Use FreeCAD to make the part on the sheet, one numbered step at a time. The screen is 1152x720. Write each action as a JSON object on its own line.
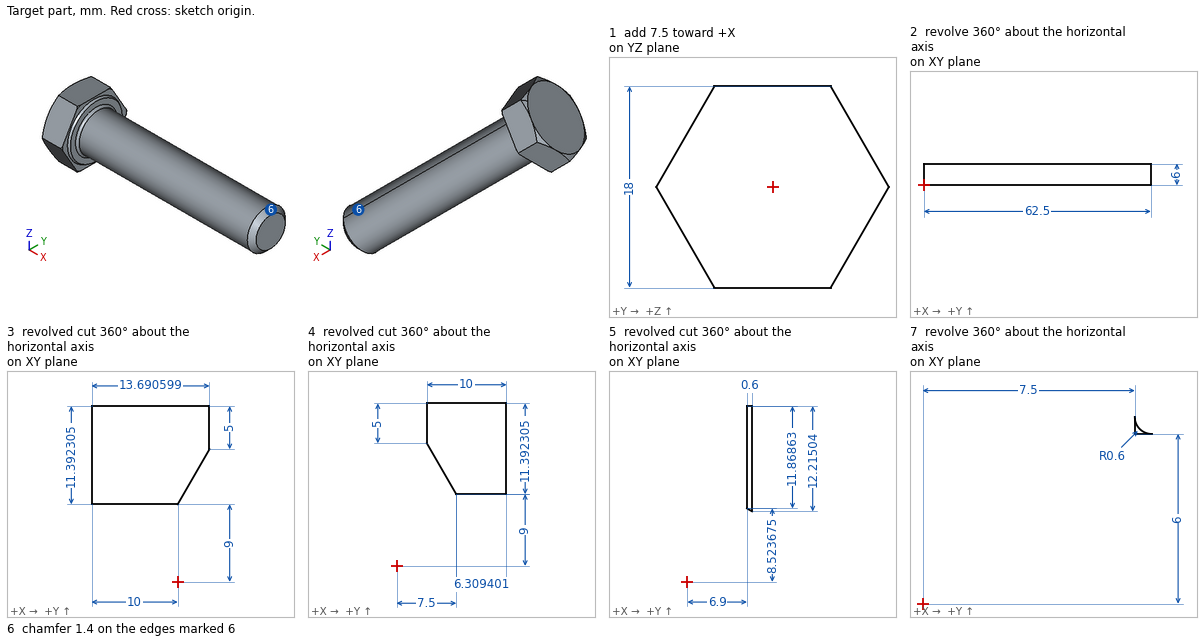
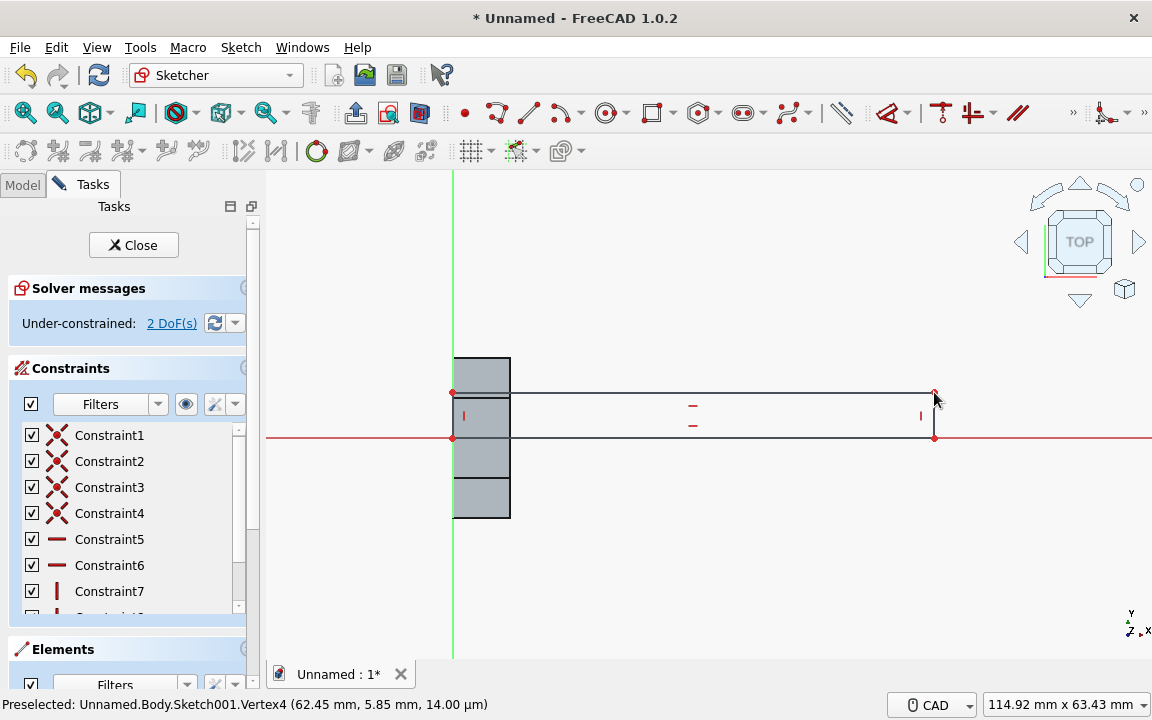
{"action": "key", "text": "d"}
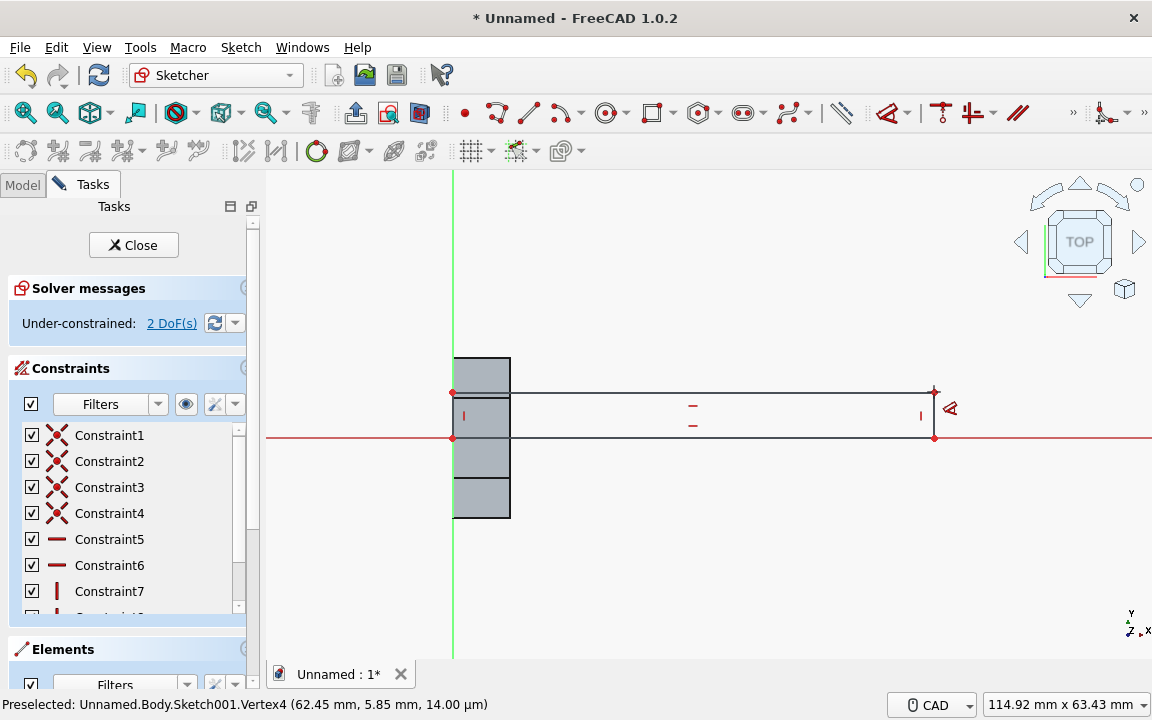
{"action": "left_click", "coordinate": [934, 425]}
{"action": "left_click", "coordinate": [968, 416]}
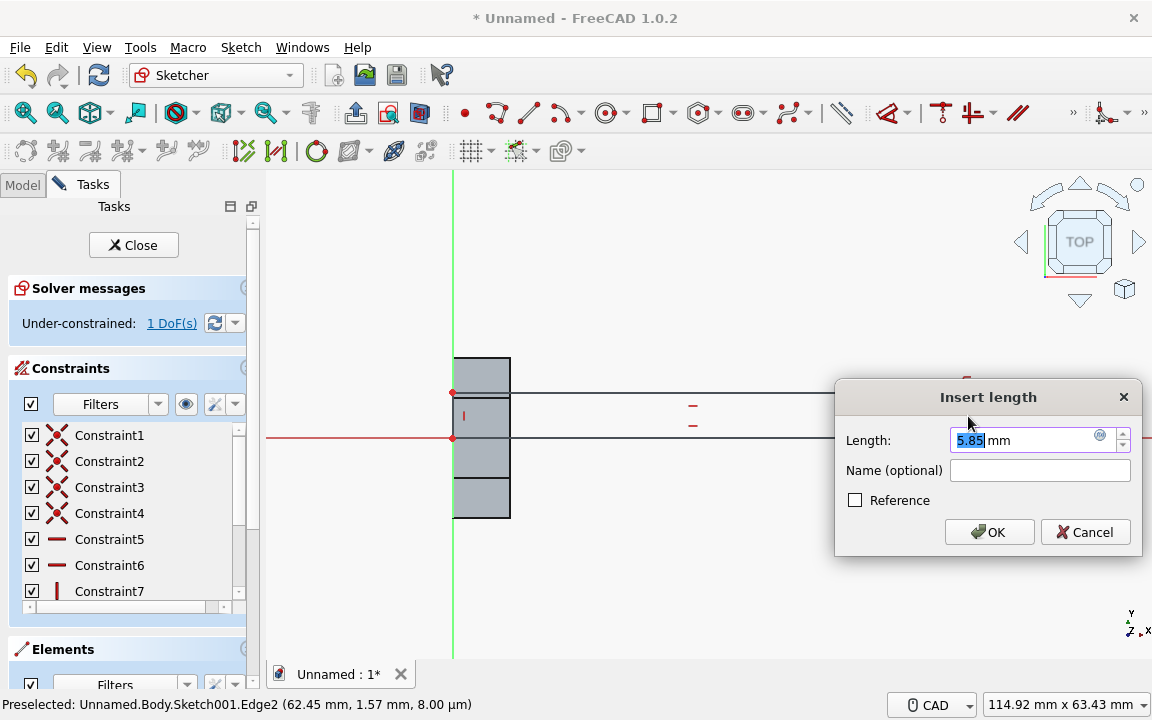
{"action": "type", "text": "6"}
{"action": "key", "text": "Return"}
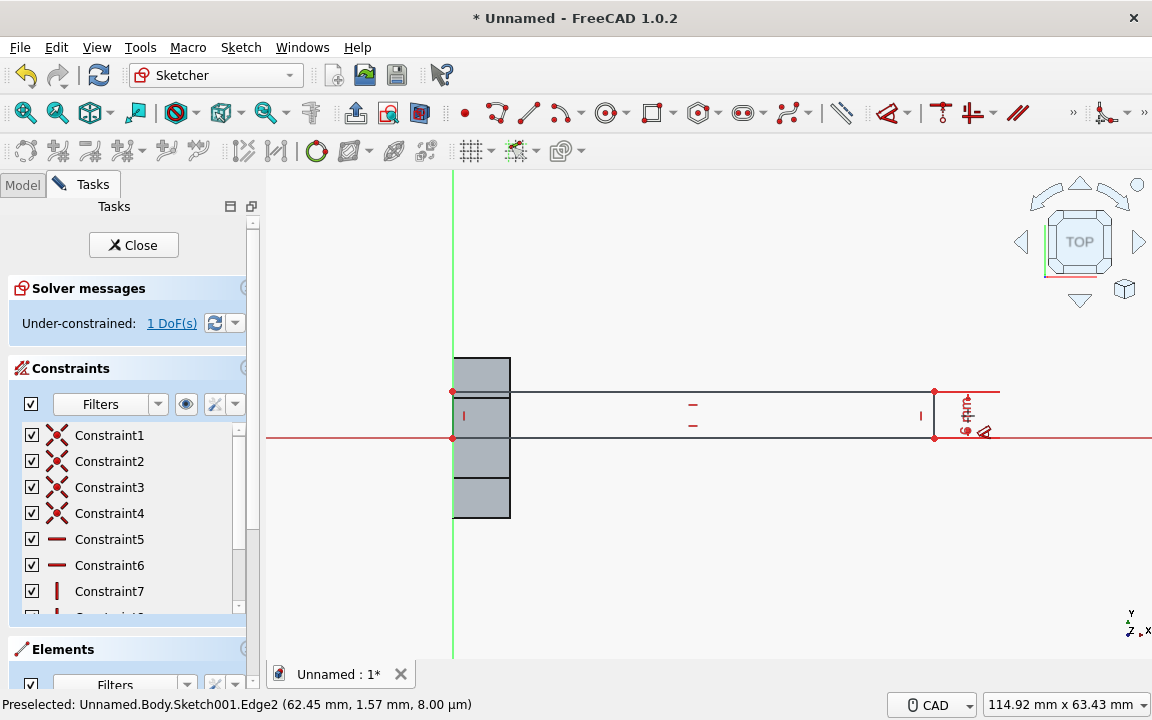
{"action": "left_click", "coordinate": [597, 438]}
{"action": "left_click", "coordinate": [693, 472]}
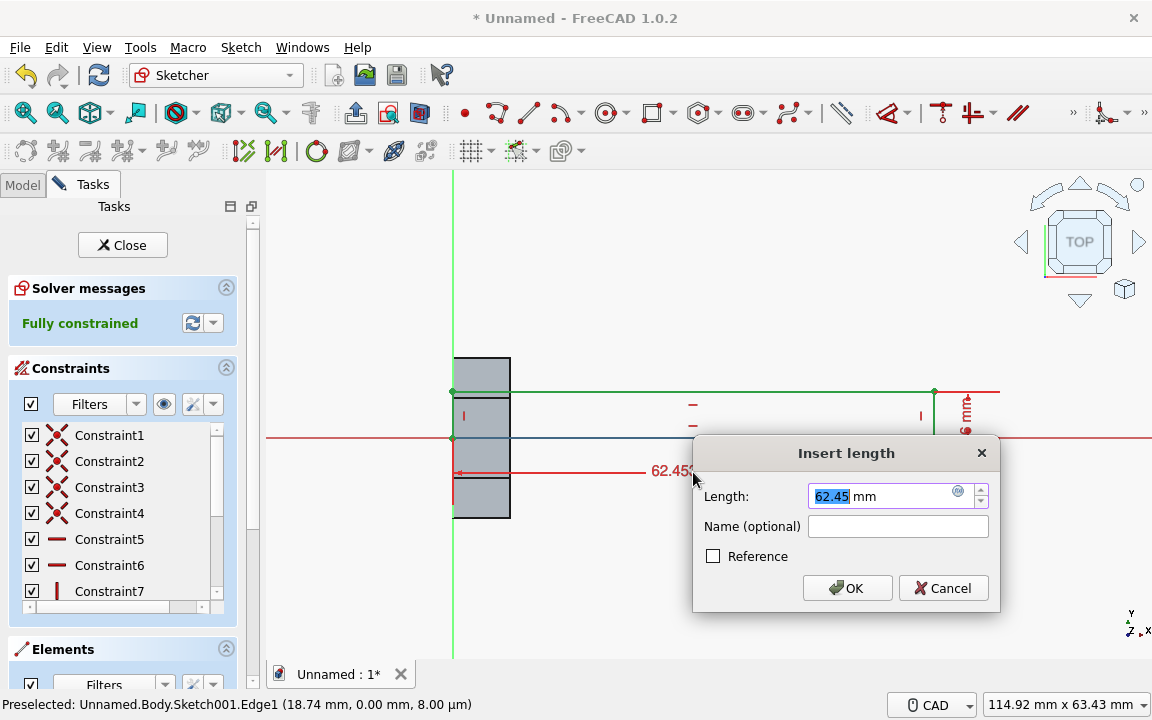
{"action": "type", "text": "62.5"}
{"action": "key", "text": "Return"}
{"action": "key", "text": "Escape"}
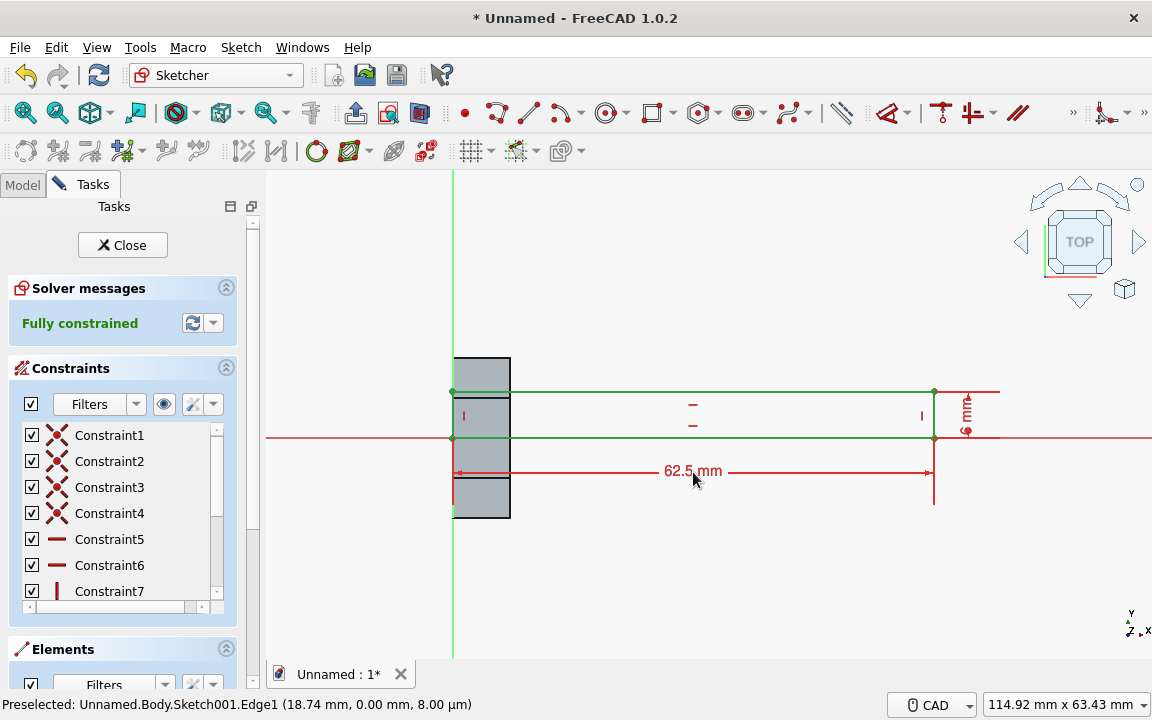
{"action": "left_click", "coordinate": [123, 245]}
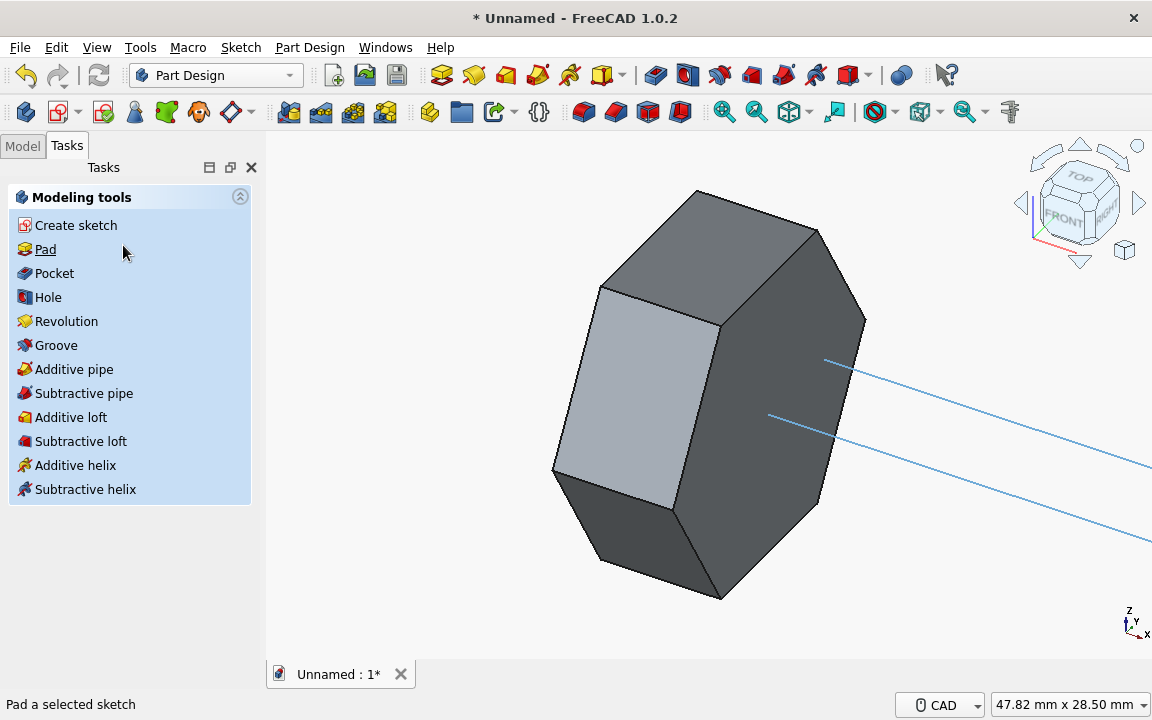
{"action": "left_click", "coordinate": [474, 76]}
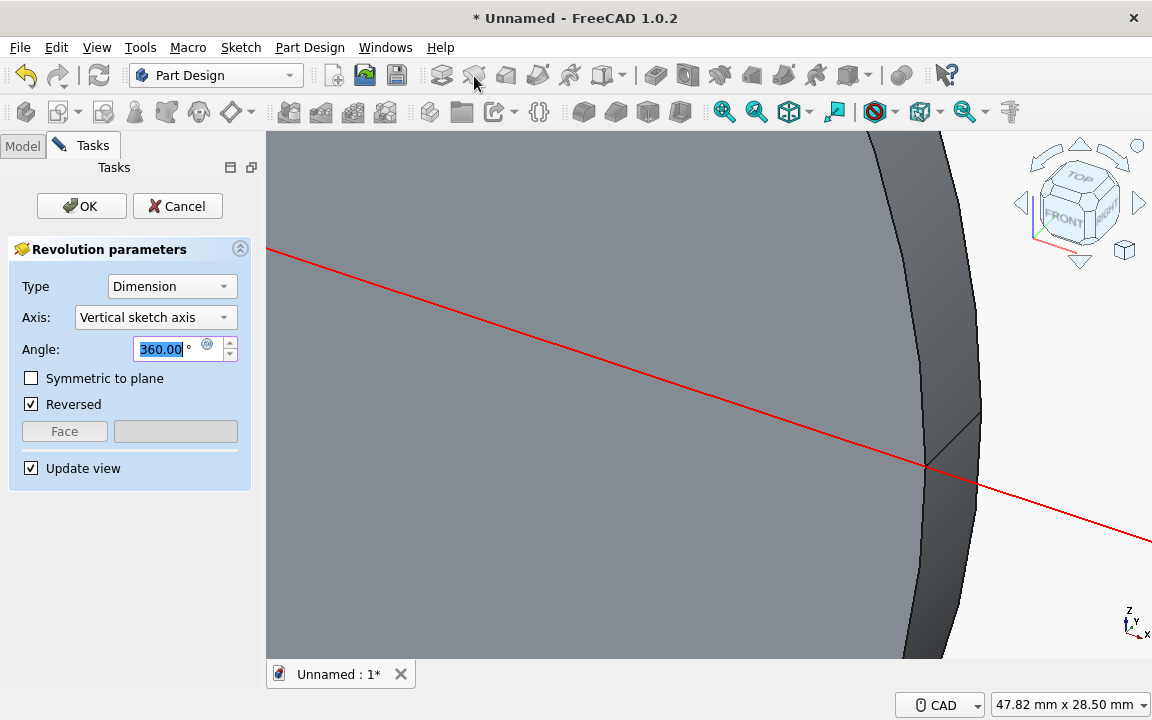
{"action": "left_click", "coordinate": [156, 318]}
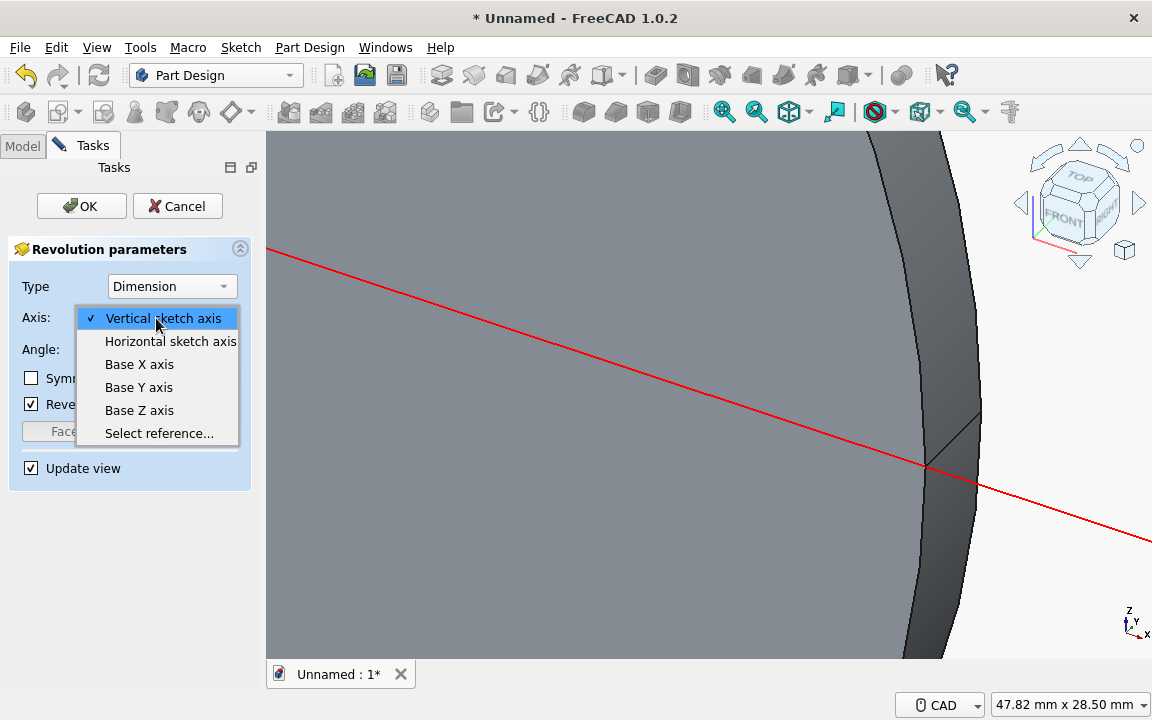
{"action": "left_click", "coordinate": [156, 342]}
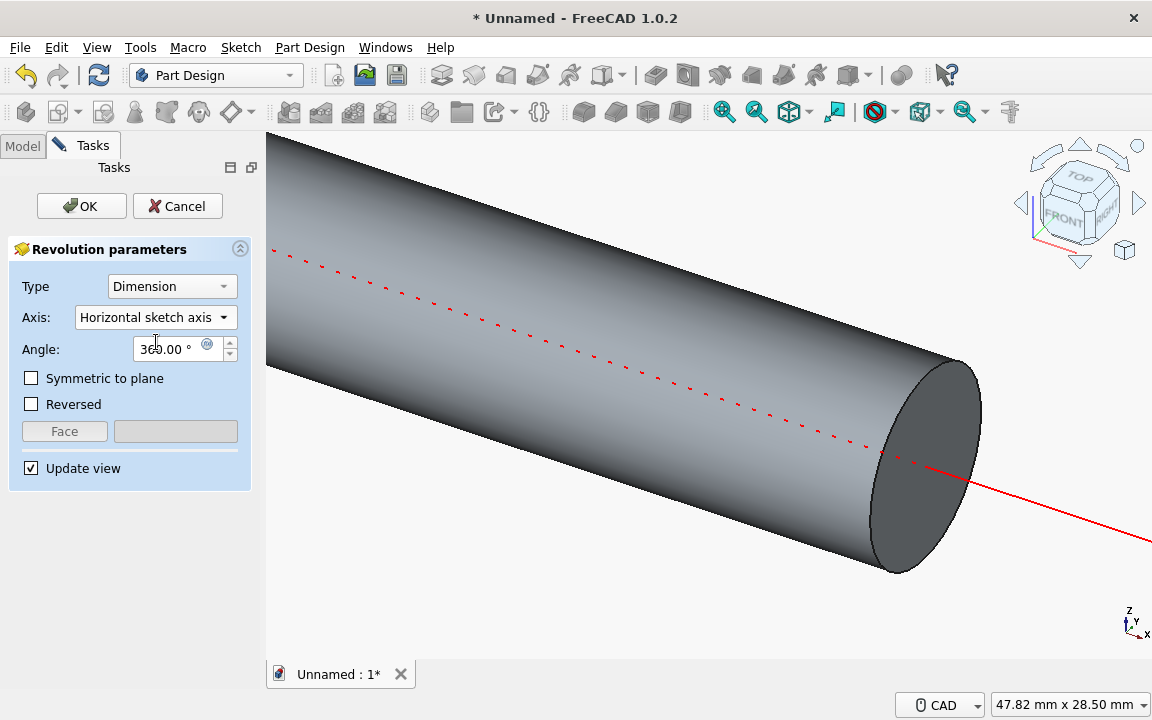
{"action": "left_click", "coordinate": [82, 206]}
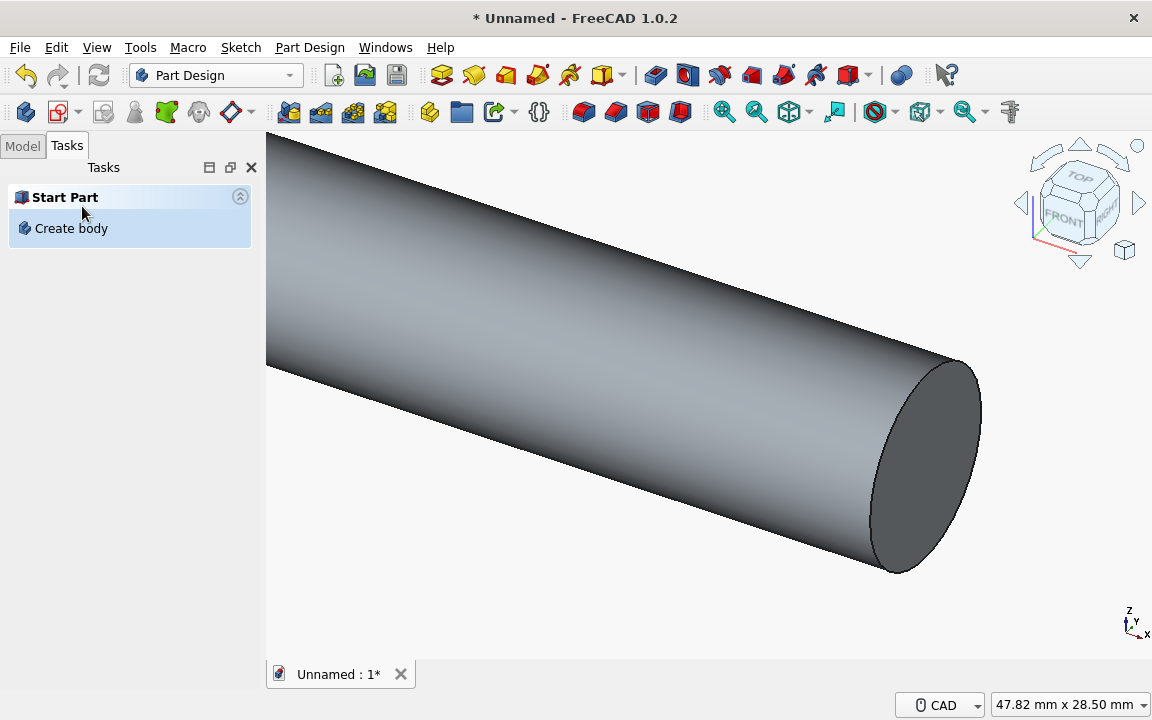
{"action": "key", "text": "v f"}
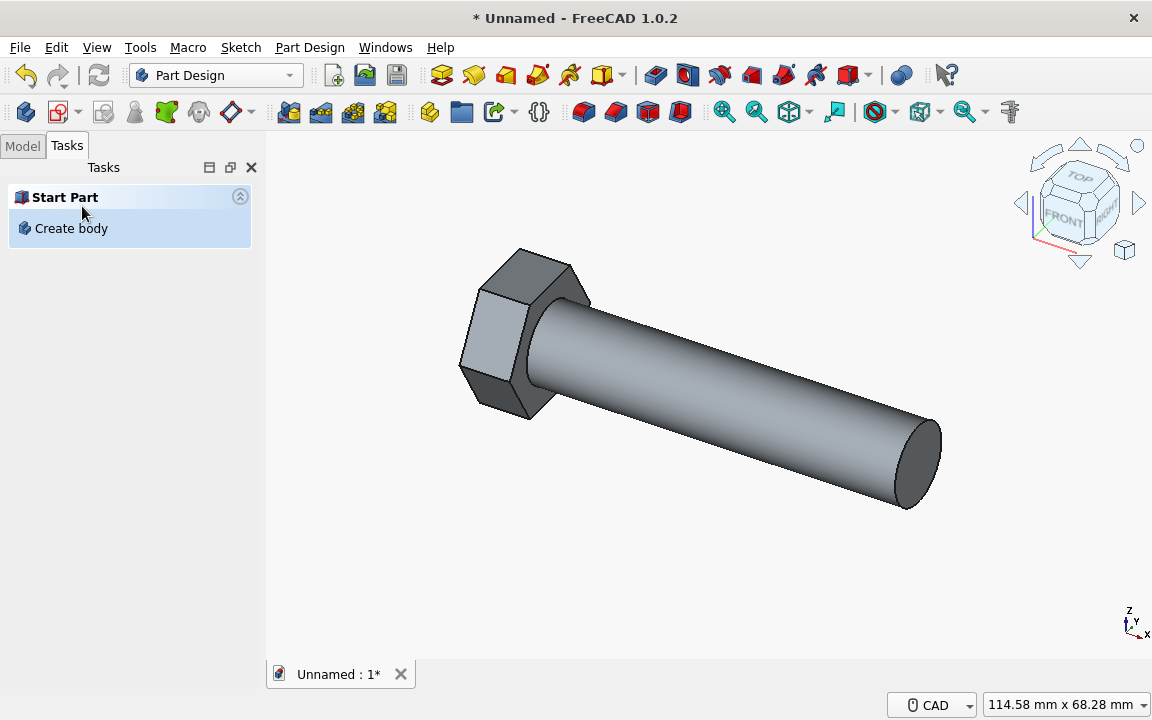
{"action": "left_click", "coordinate": [58, 112]}